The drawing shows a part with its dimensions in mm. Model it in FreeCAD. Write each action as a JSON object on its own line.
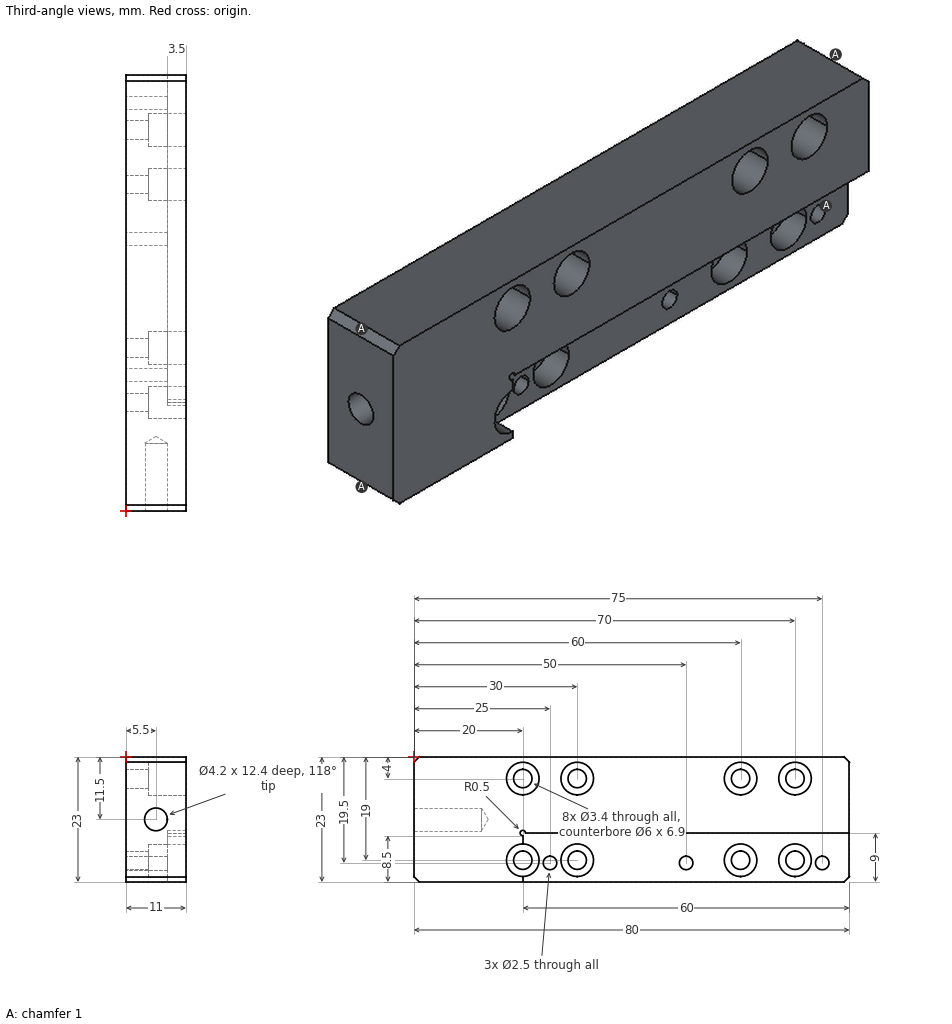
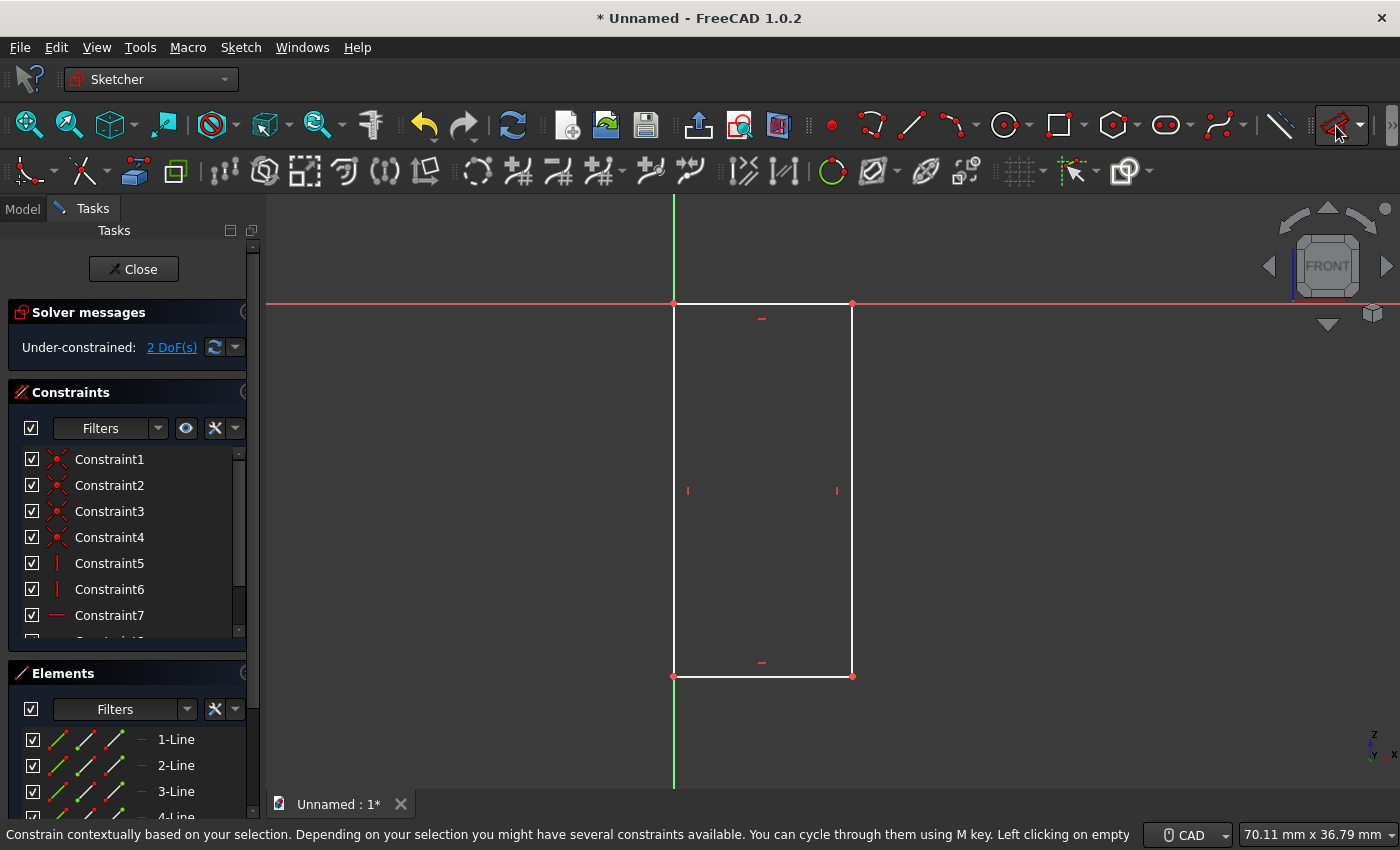
{"action": "left_click", "coordinate": [674, 416]}
{"action": "left_click", "coordinate": [640, 490]}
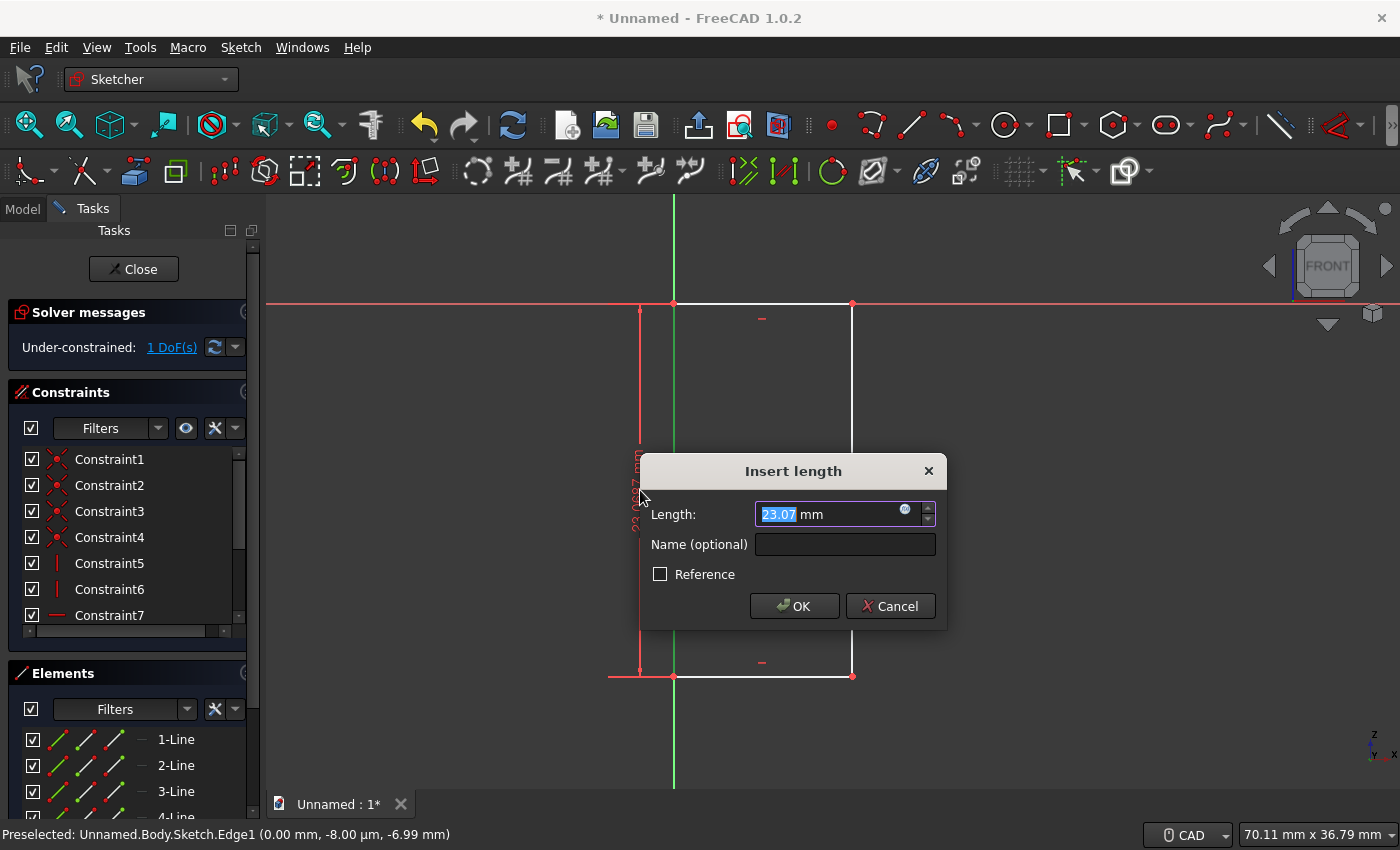
{"action": "type", "text": "23"}
{"action": "key", "text": "Return"}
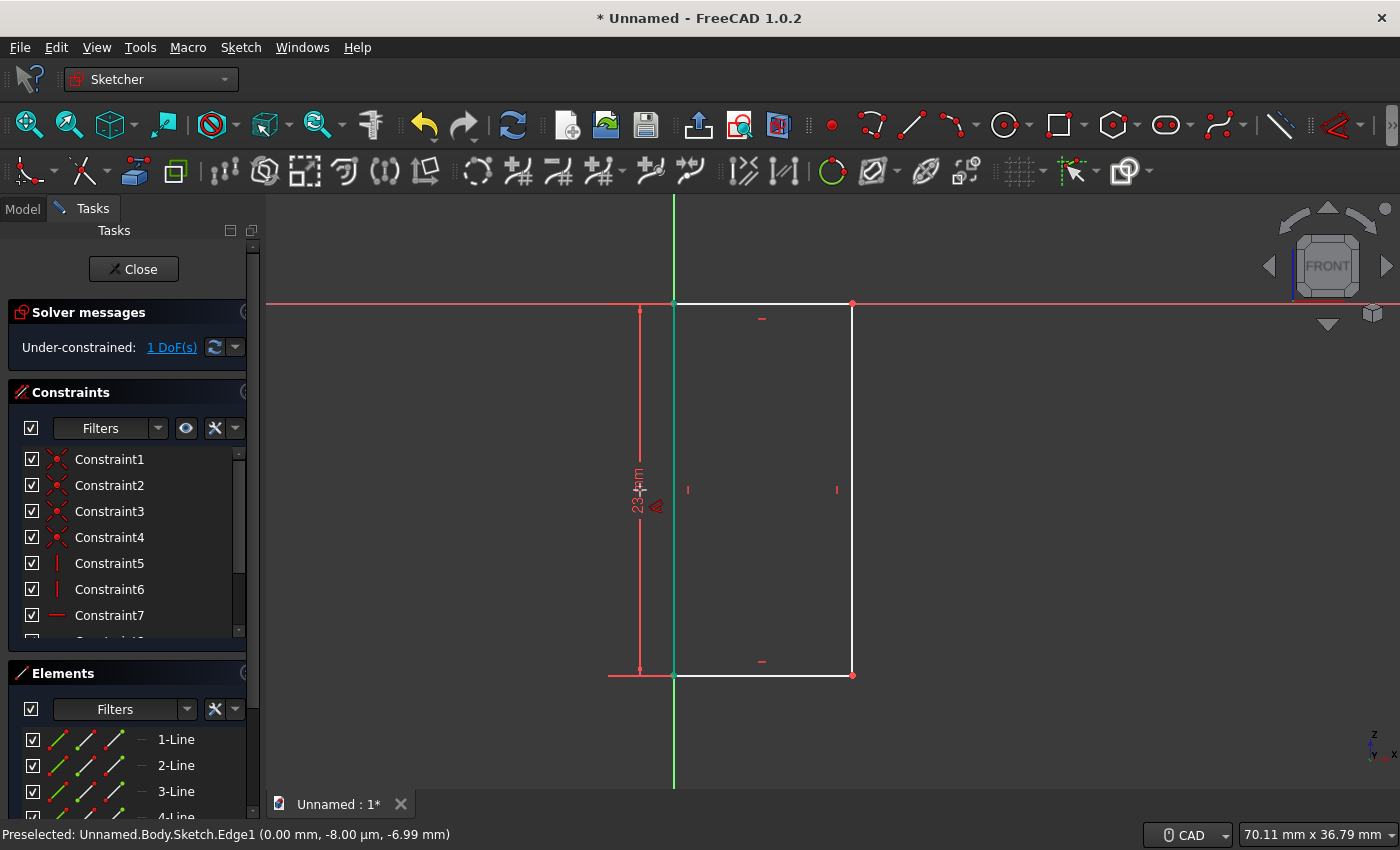
{"action": "left_click", "coordinate": [727, 676]}
{"action": "left_click", "coordinate": [763, 710]}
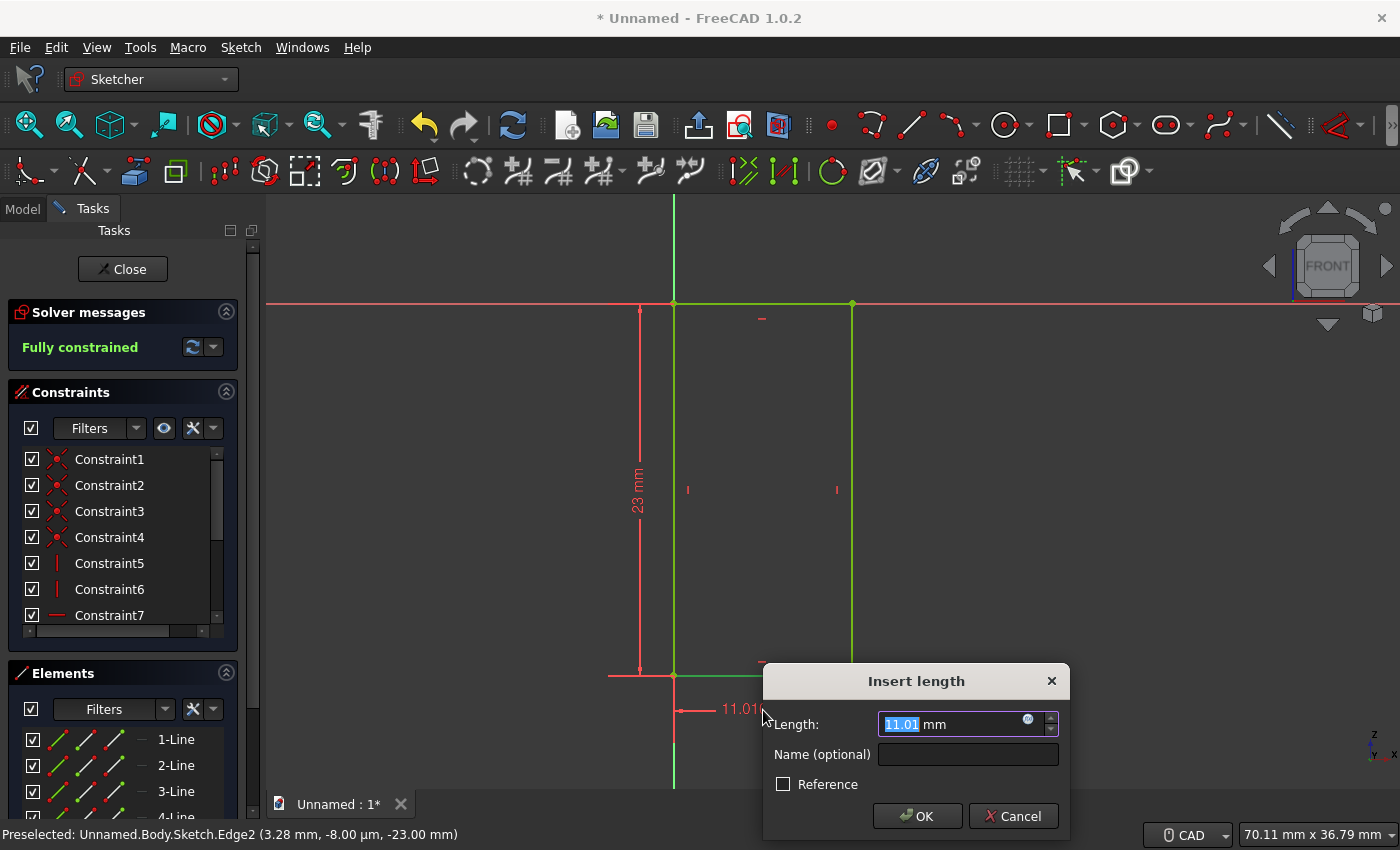
{"action": "type", "text": "11"}
{"action": "key", "text": "Return"}
{"action": "key", "text": "Escape"}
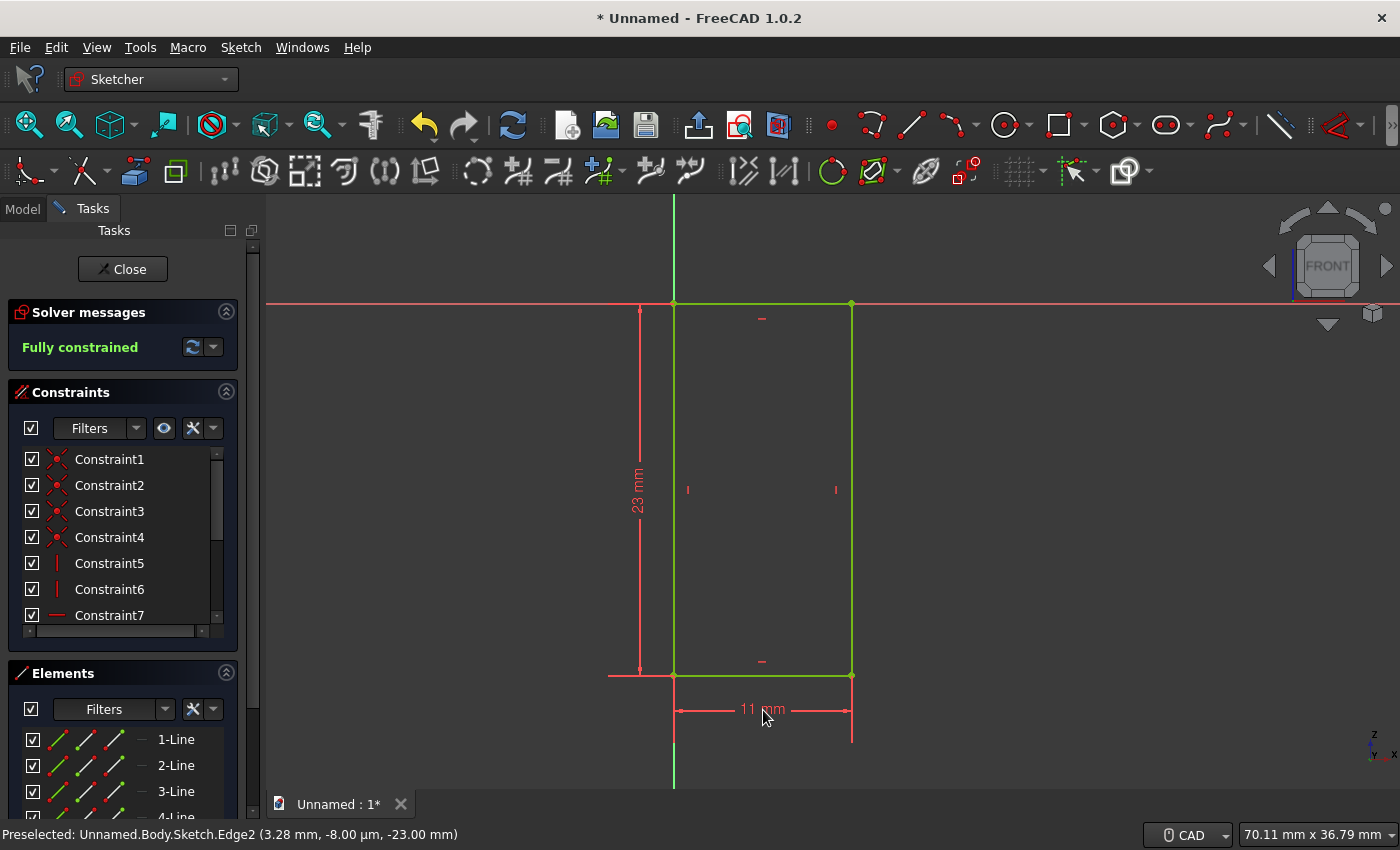
{"action": "left_click", "coordinate": [123, 269]}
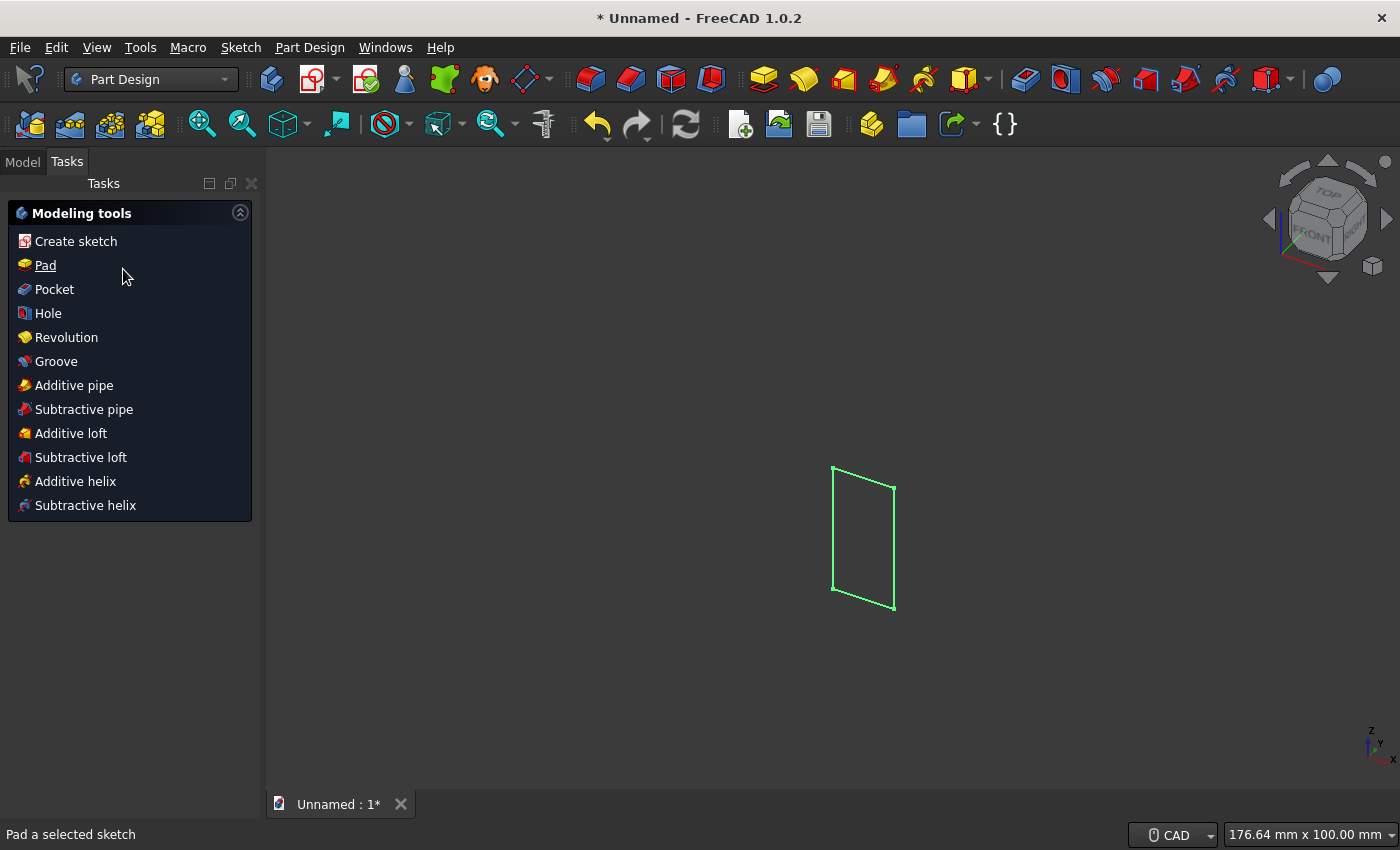
{"action": "left_click", "coordinate": [764, 80]}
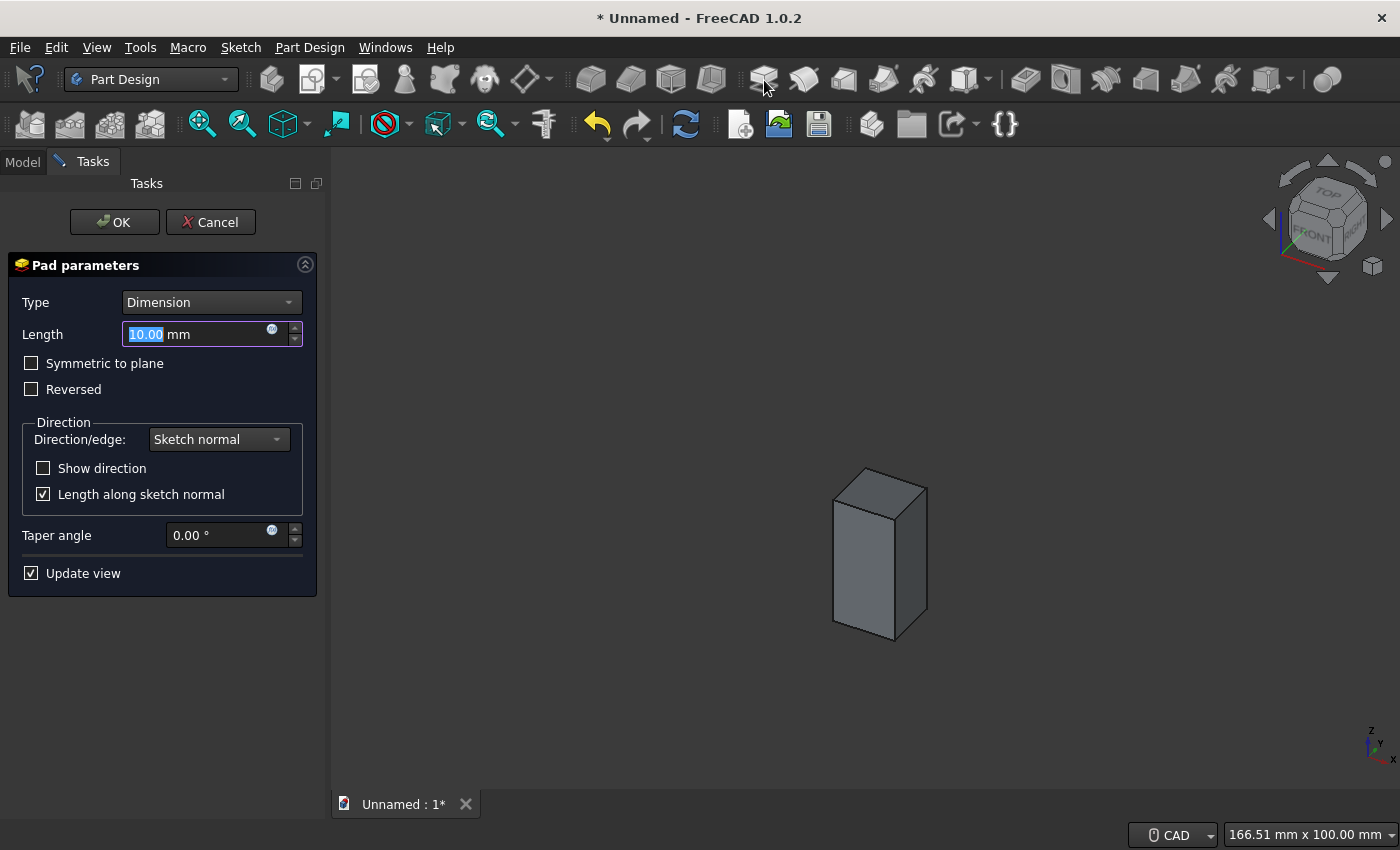
{"action": "type", "text": "80"}
{"action": "key", "text": "Tab"}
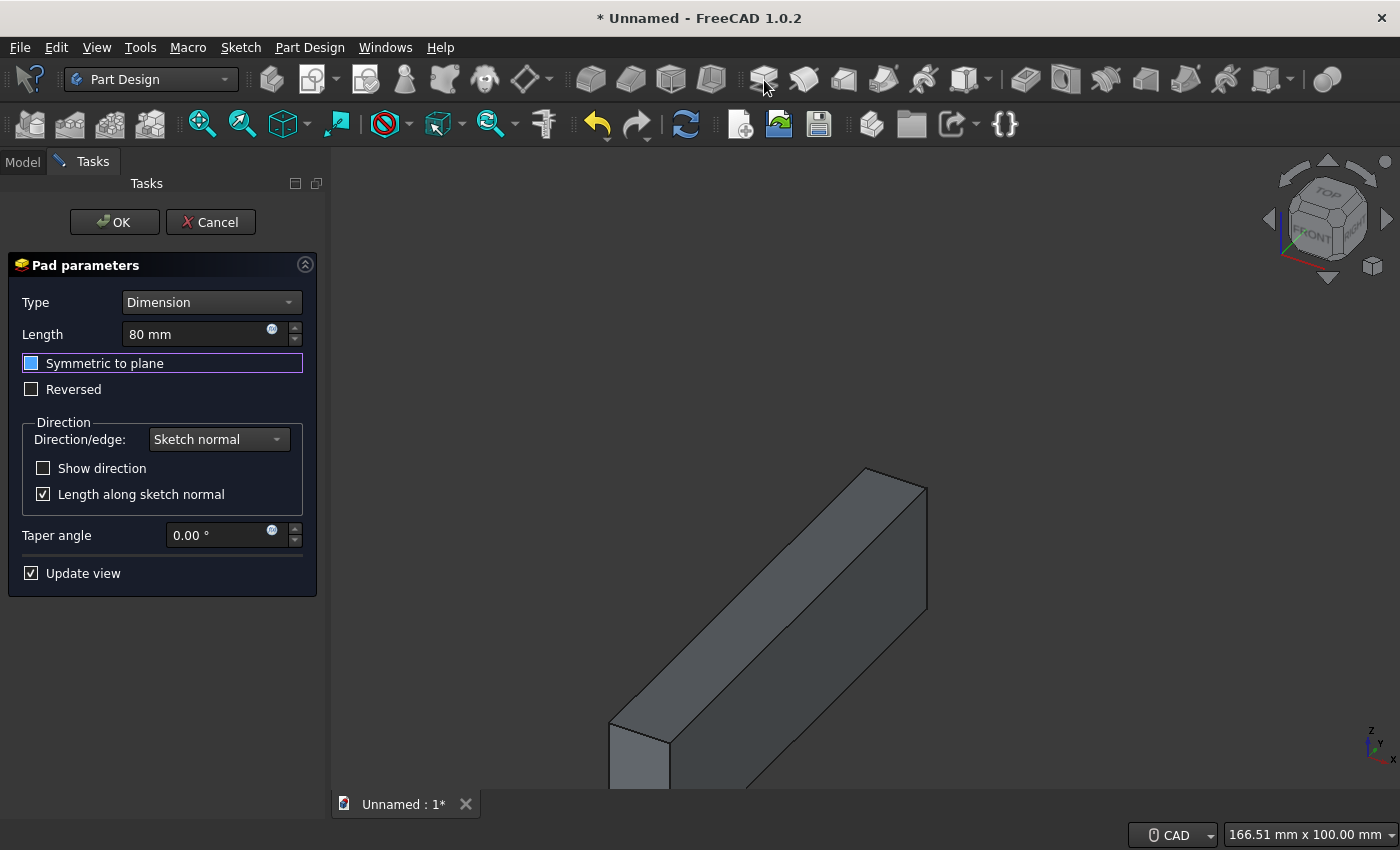
{"action": "left_click", "coordinate": [30, 389]}